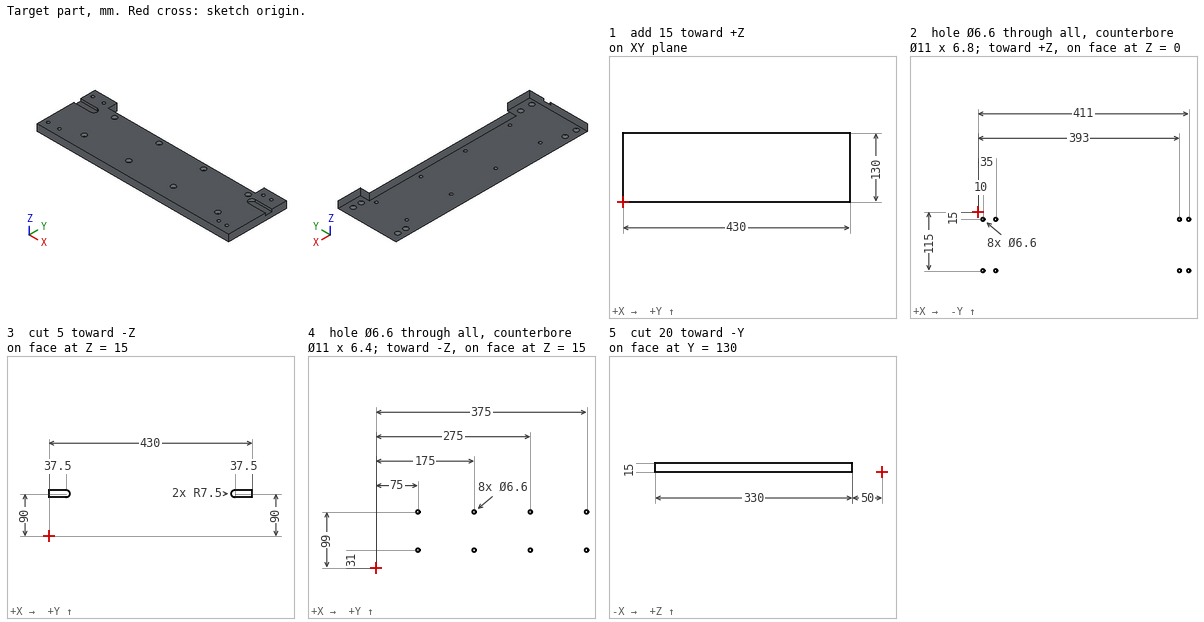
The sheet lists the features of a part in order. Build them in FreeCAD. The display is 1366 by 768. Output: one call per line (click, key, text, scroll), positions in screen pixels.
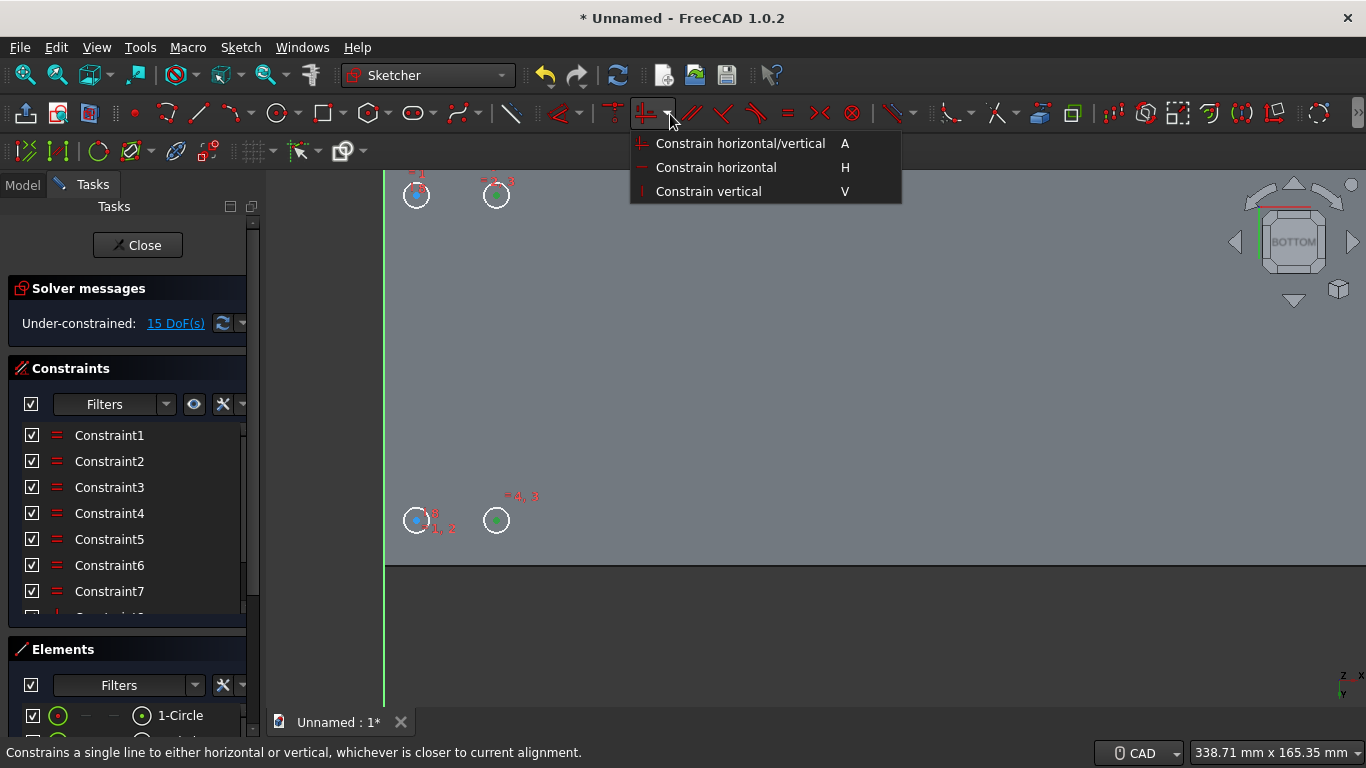
click(766, 191)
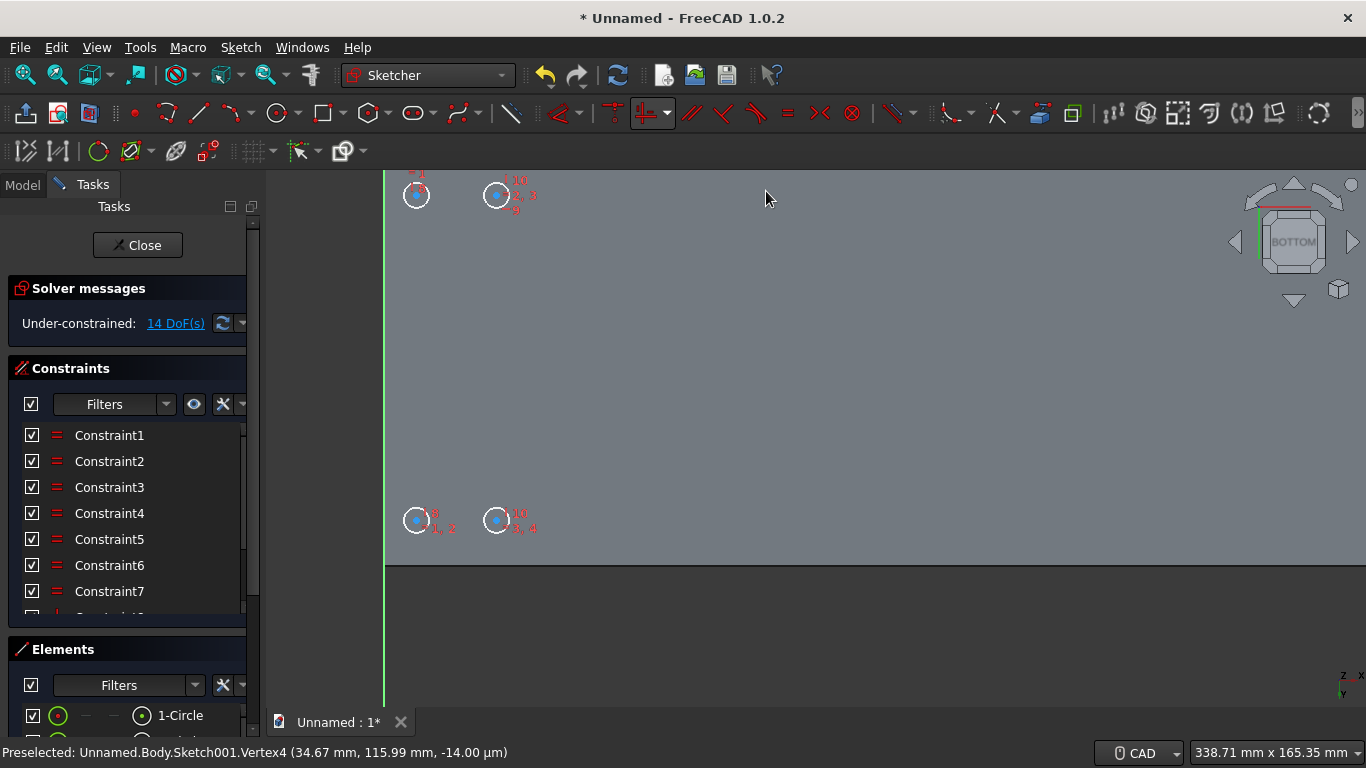
click(416, 520)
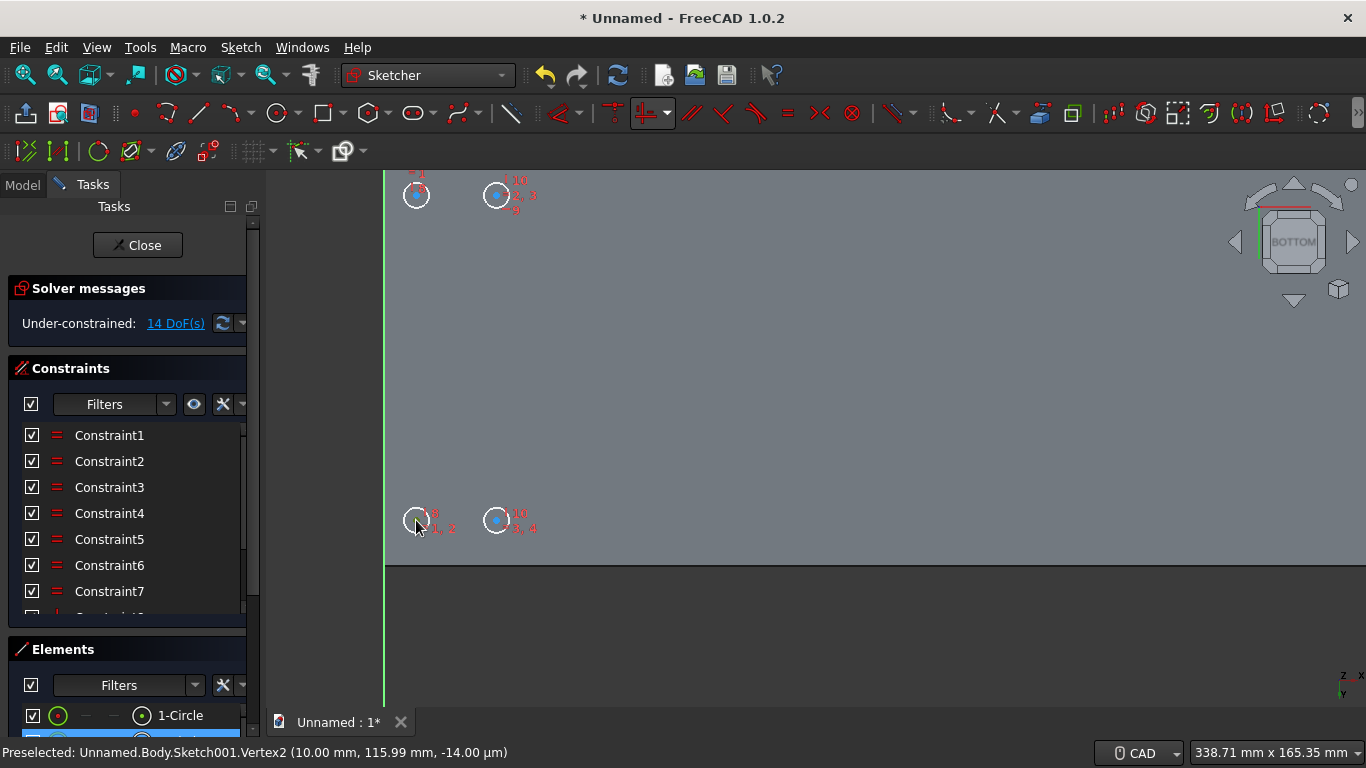
click(497, 520)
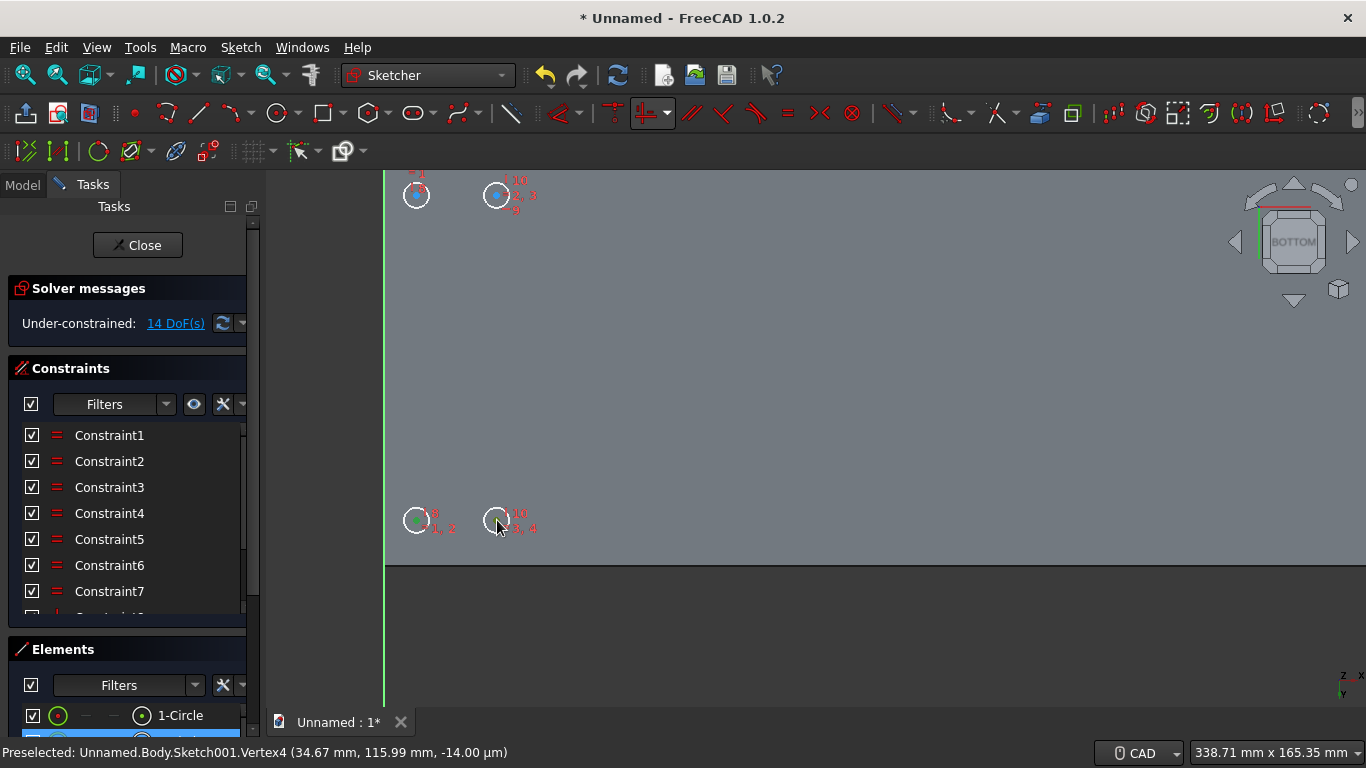
key(h)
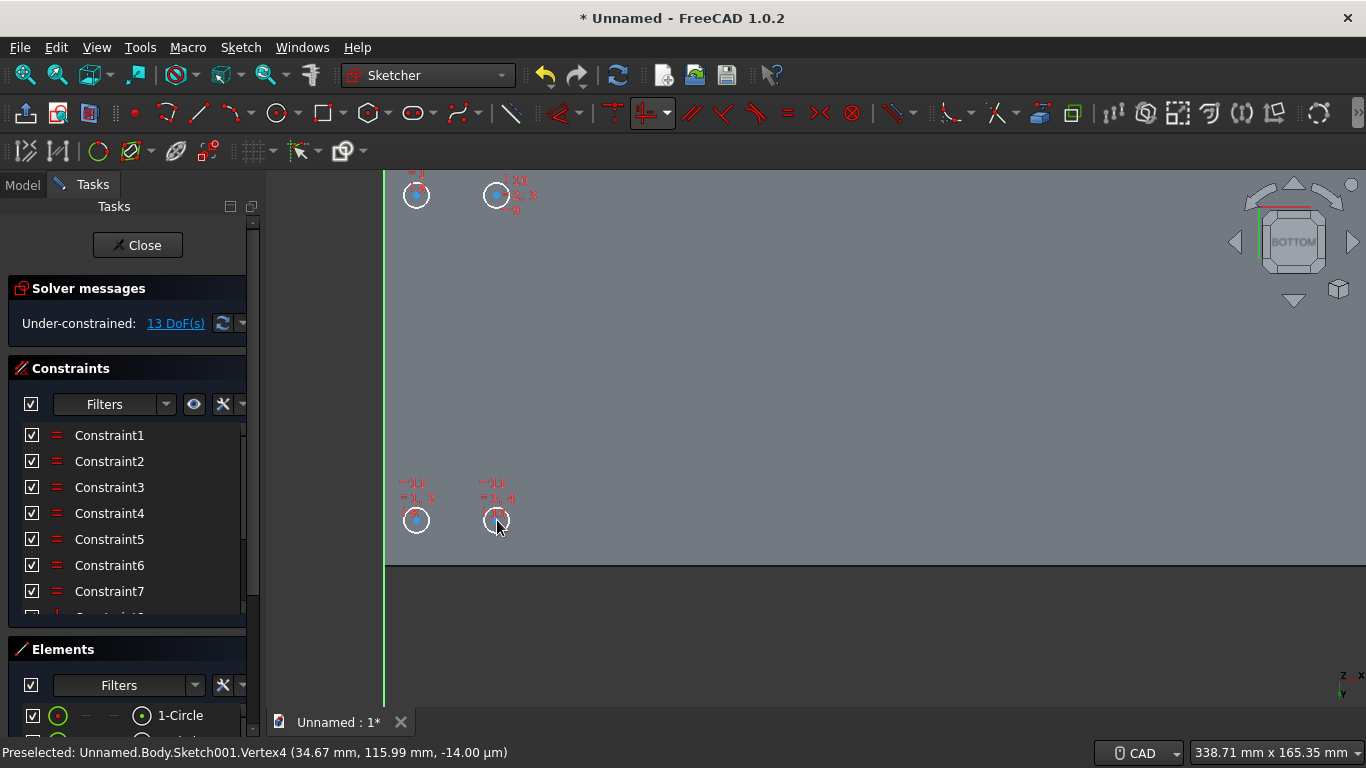
scroll(495, 522, down, 4)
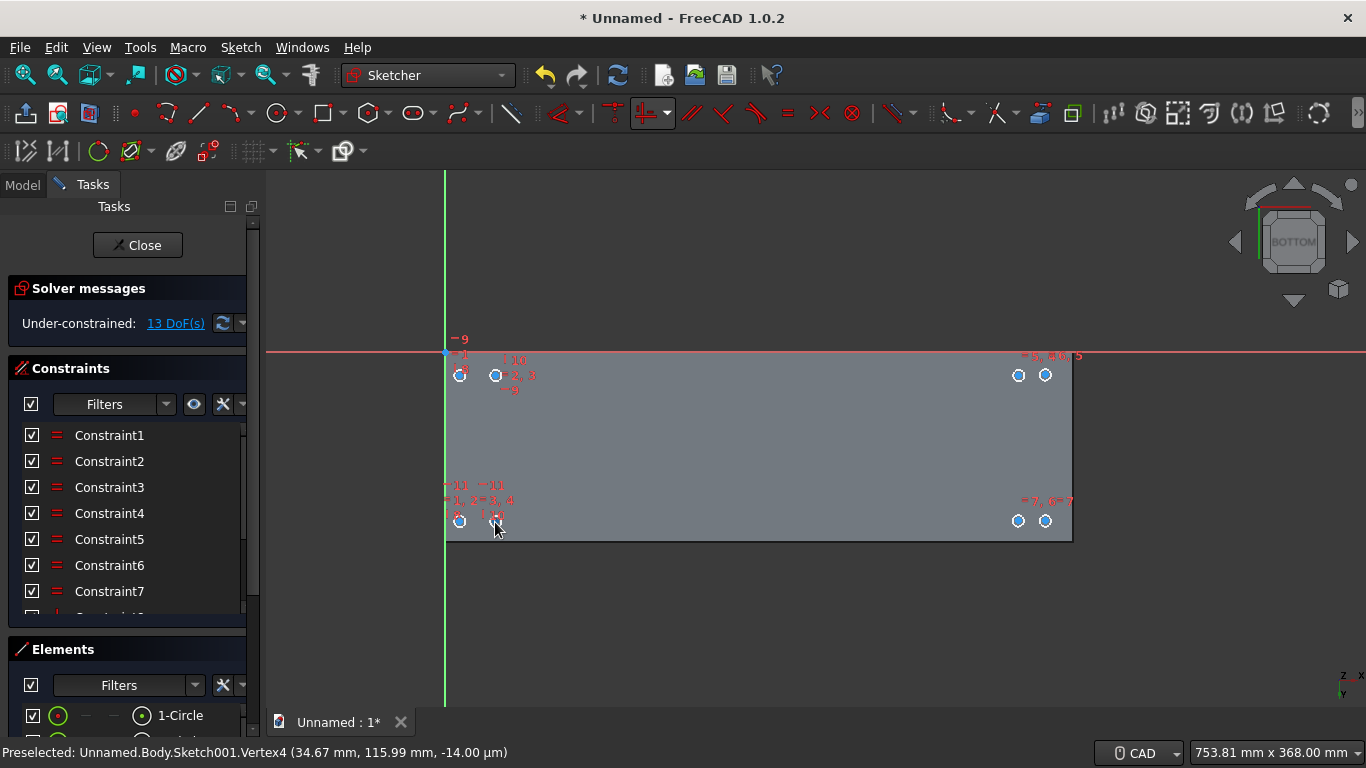
click(496, 376)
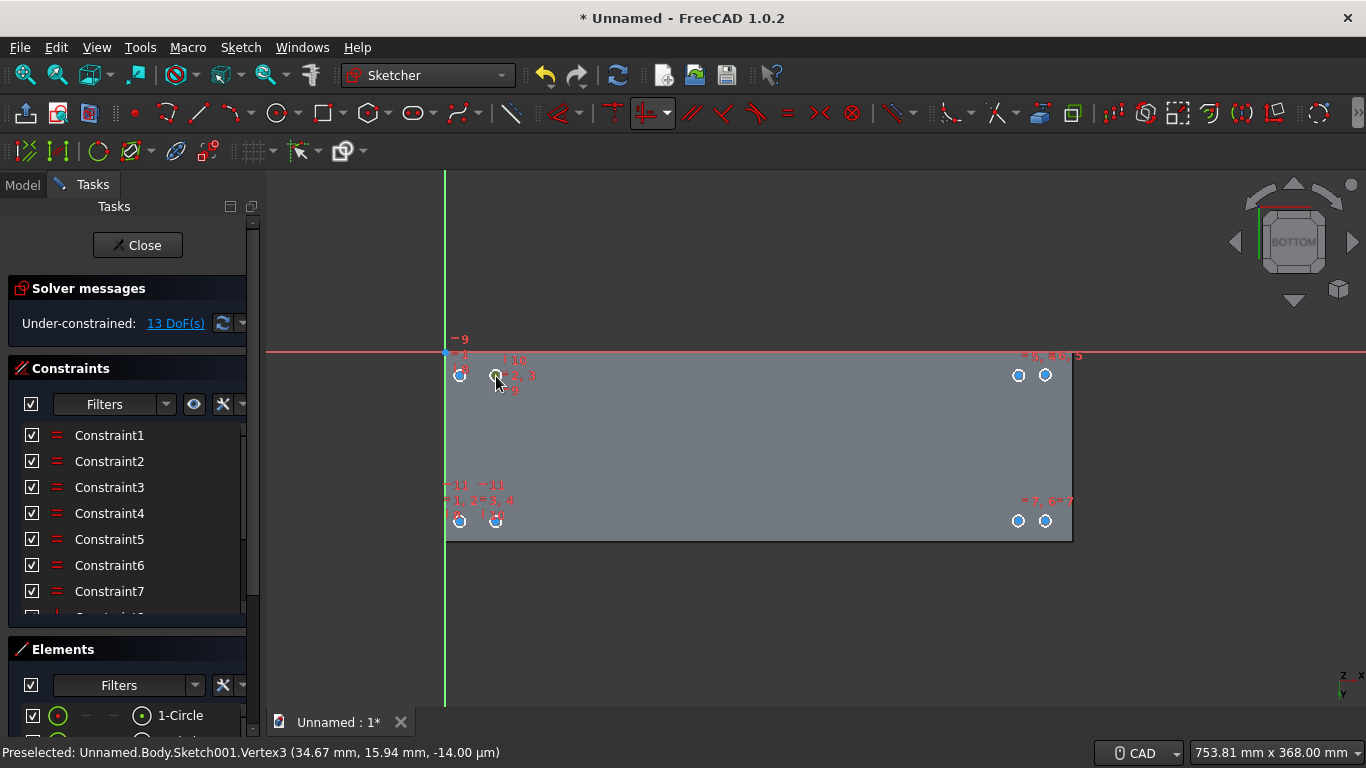
click(1019, 376)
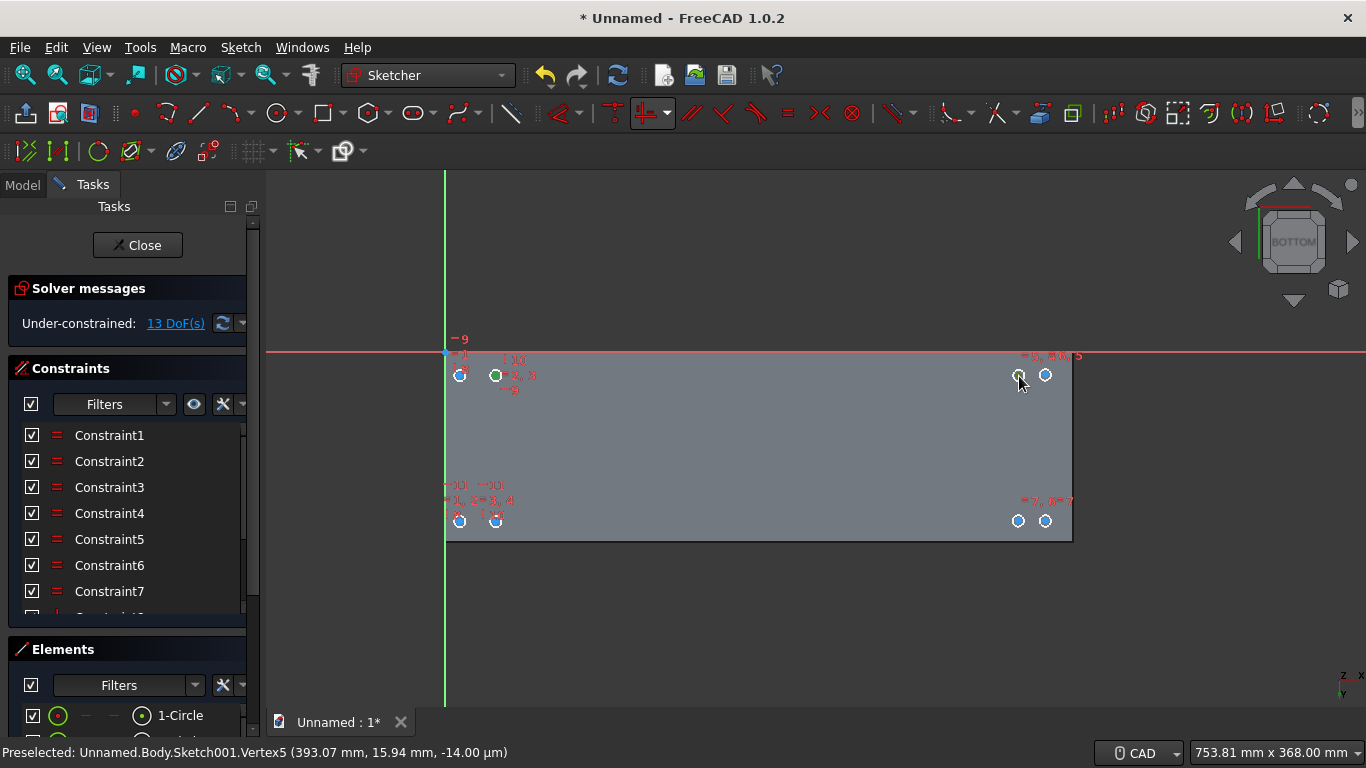
click(670, 114)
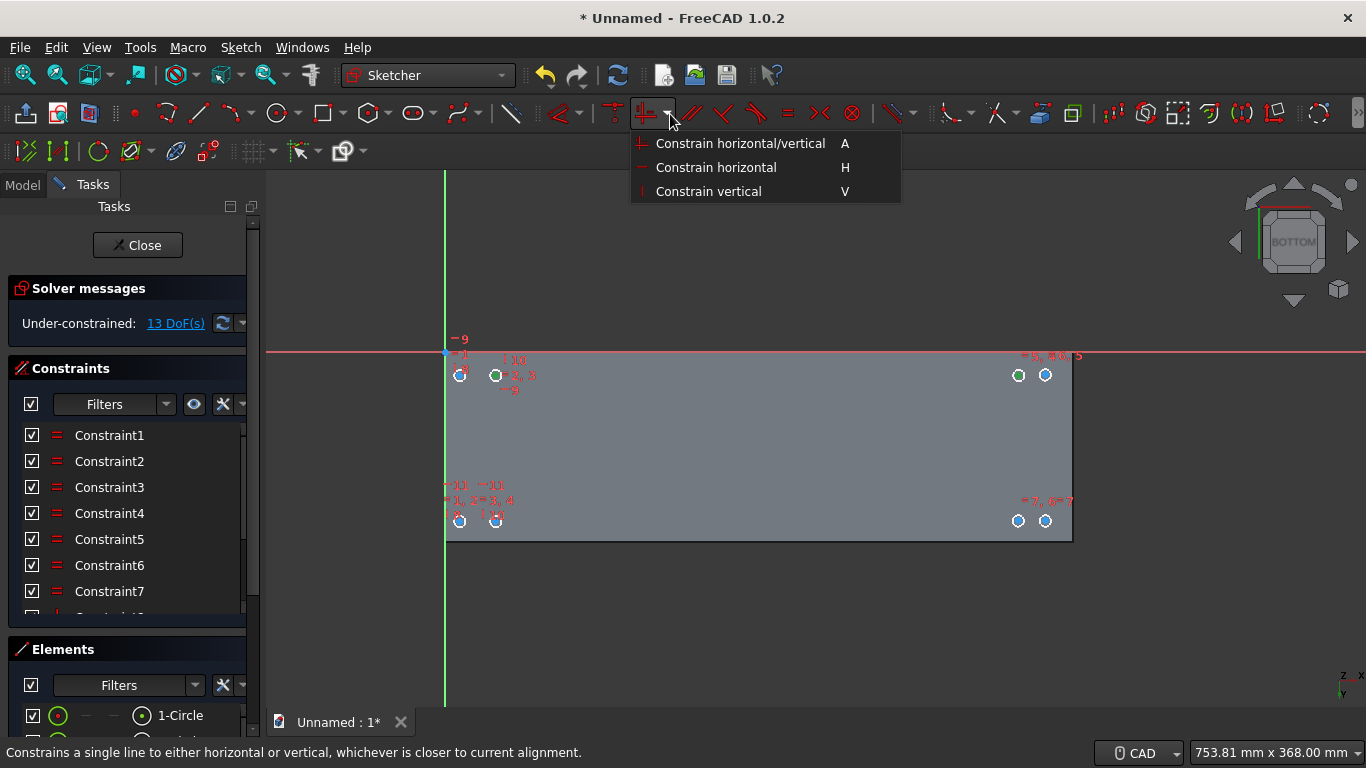
click(766, 167)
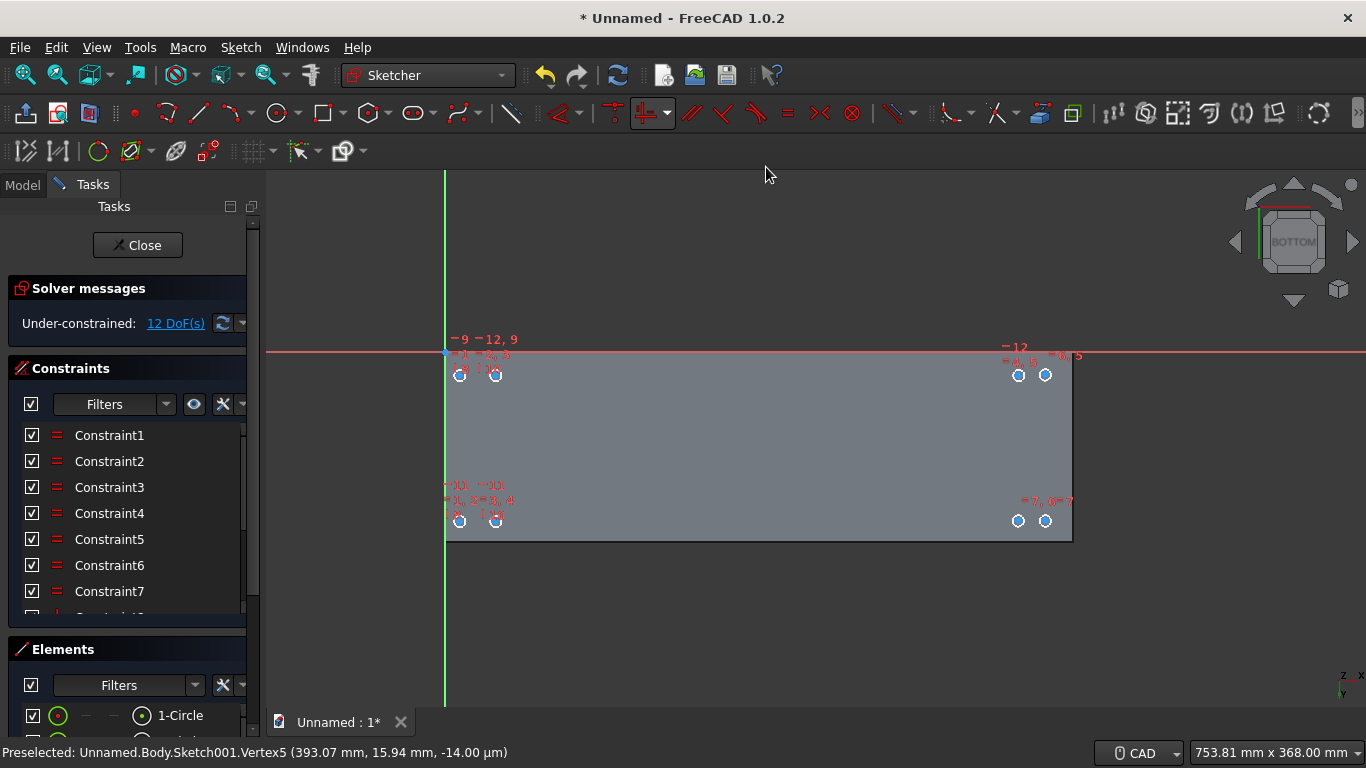
click(1019, 376)